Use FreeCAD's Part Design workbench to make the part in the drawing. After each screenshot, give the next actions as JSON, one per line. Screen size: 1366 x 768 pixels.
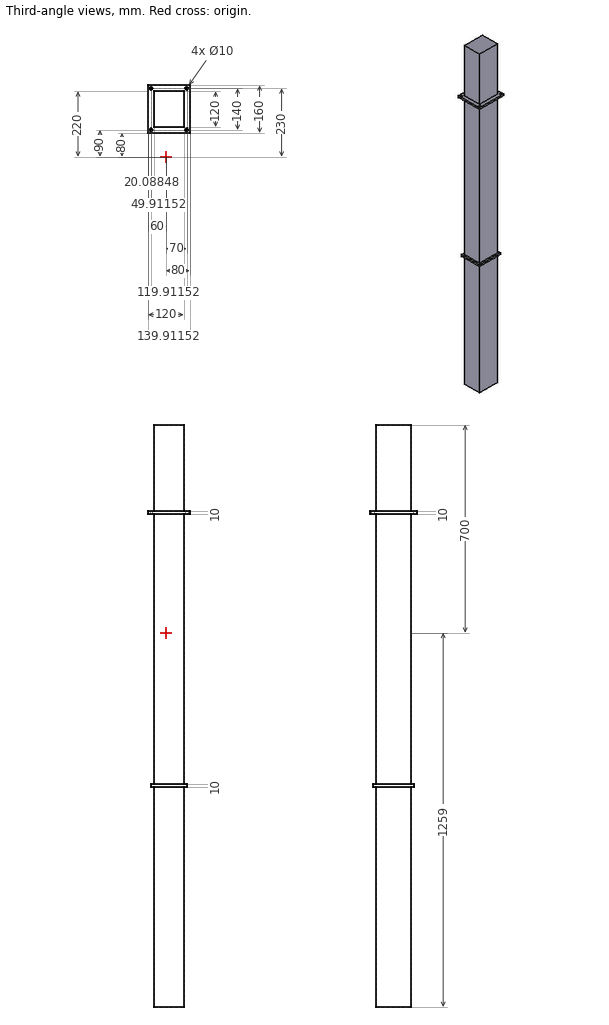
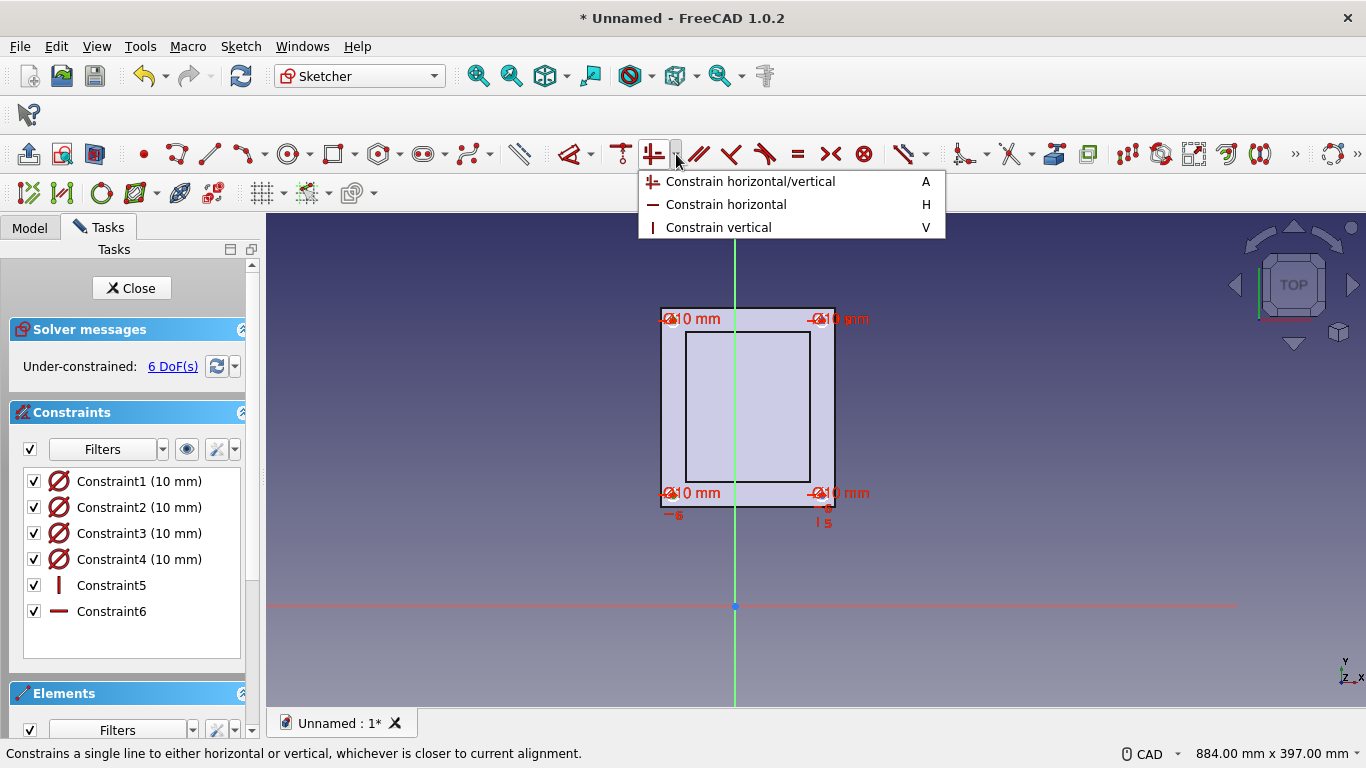
{"action": "left_click", "coordinate": [792, 228]}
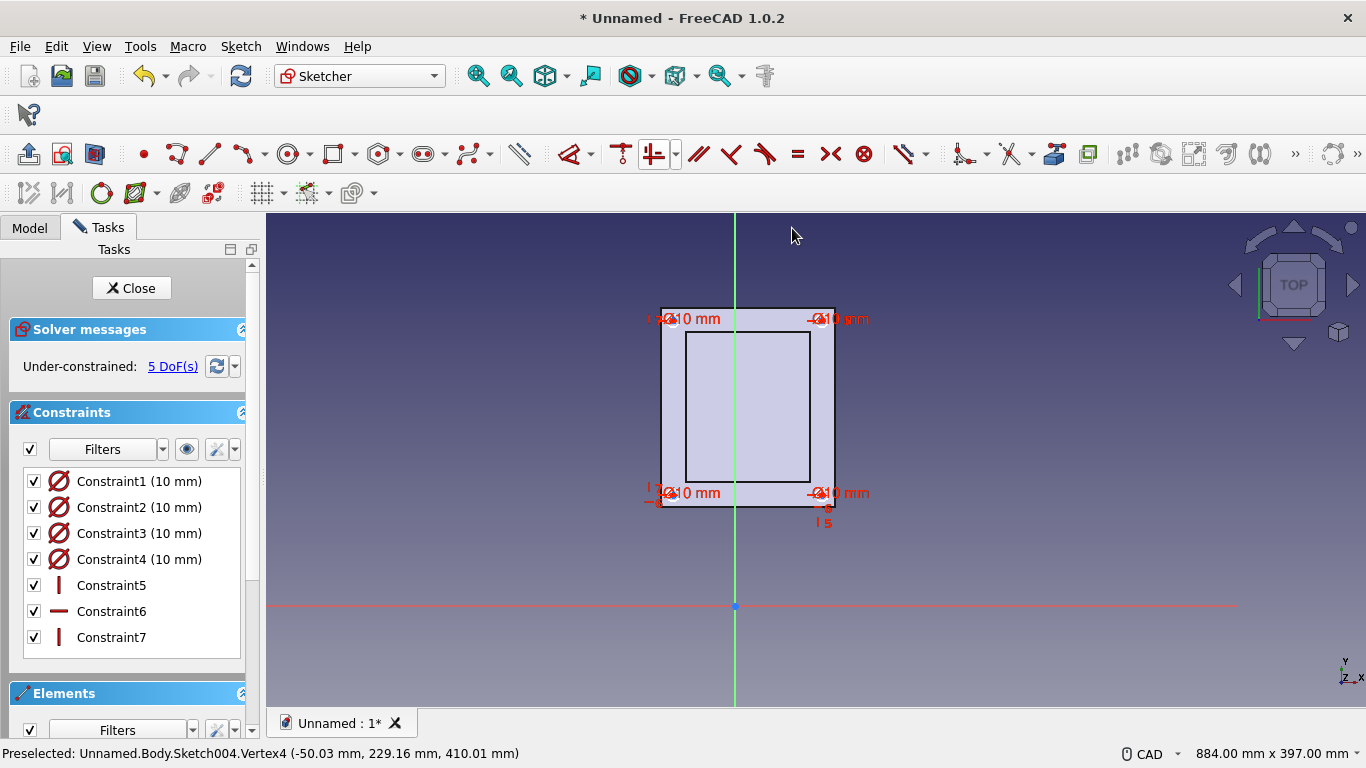
{"action": "left_click", "coordinate": [822, 321]}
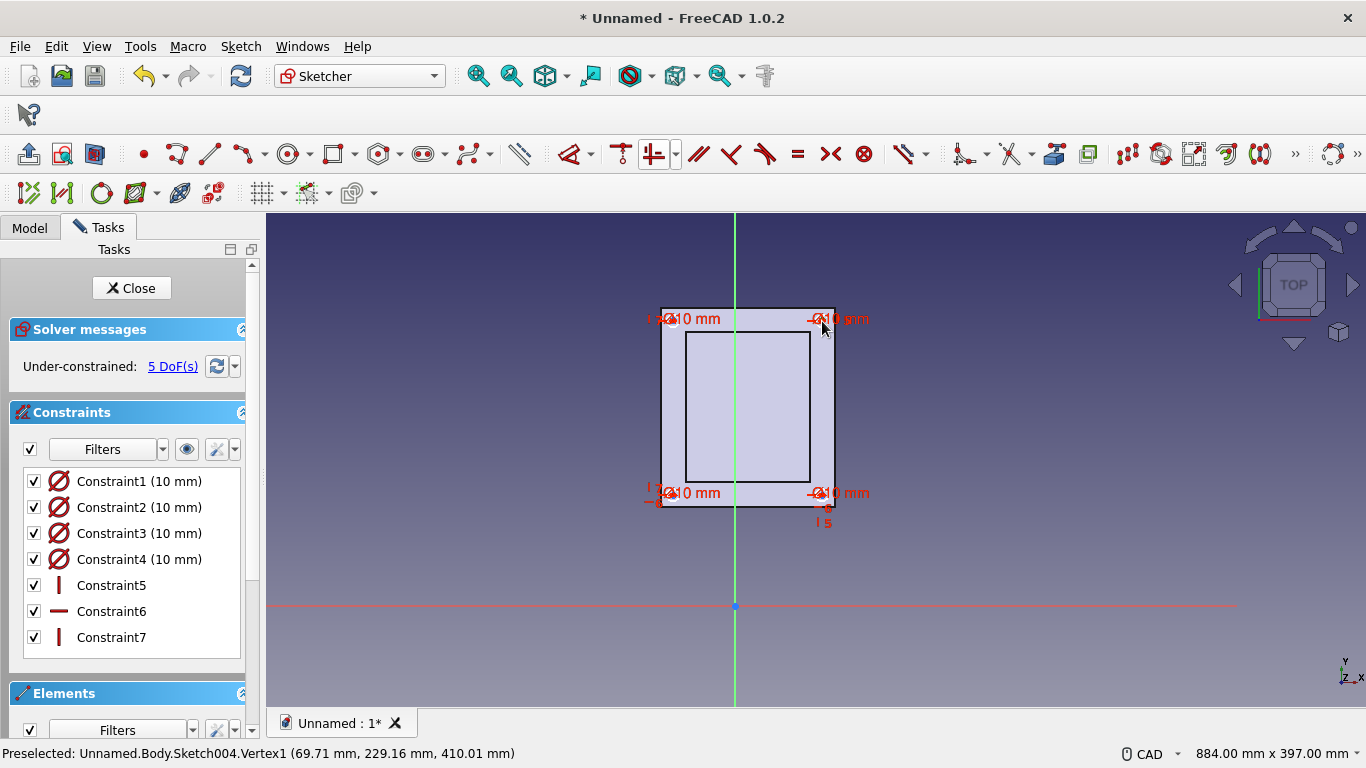
{"action": "left_click", "coordinate": [673, 321]}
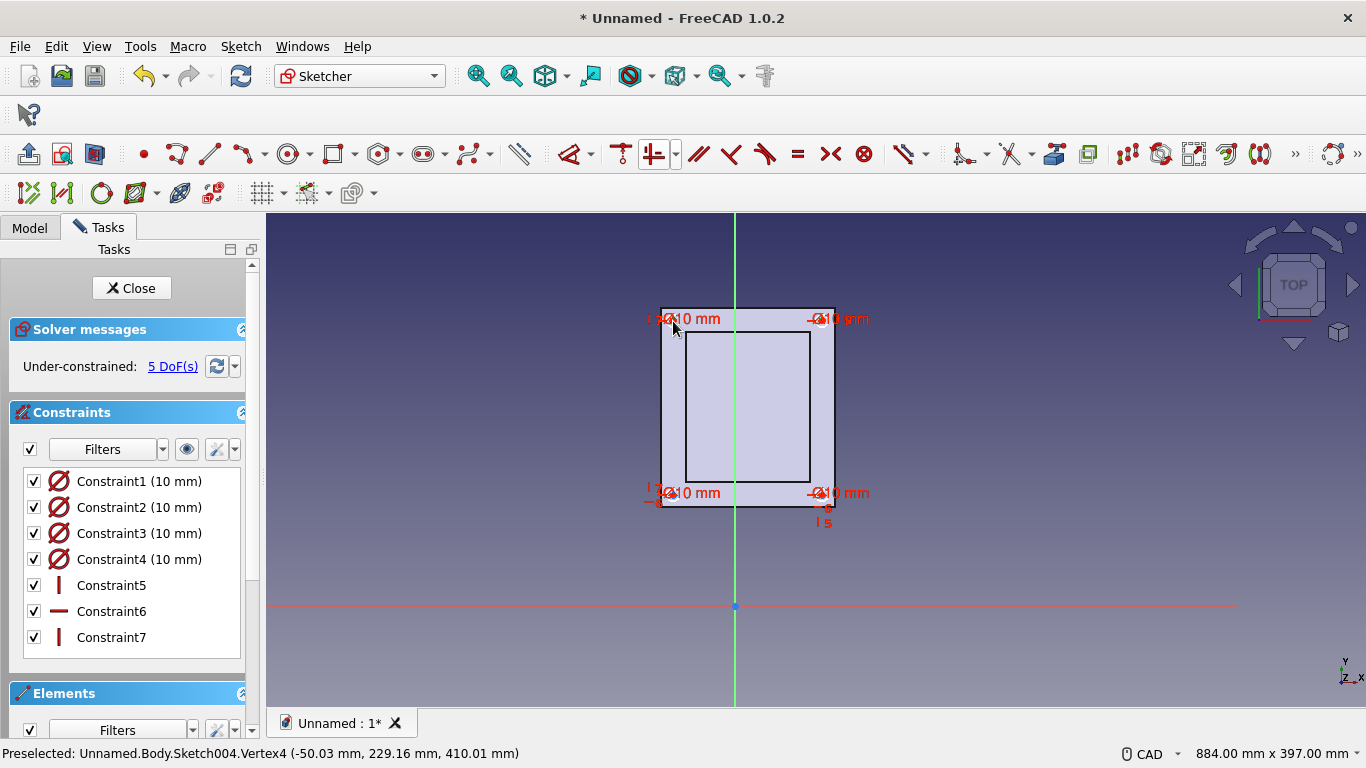
{"action": "key", "text": "h"}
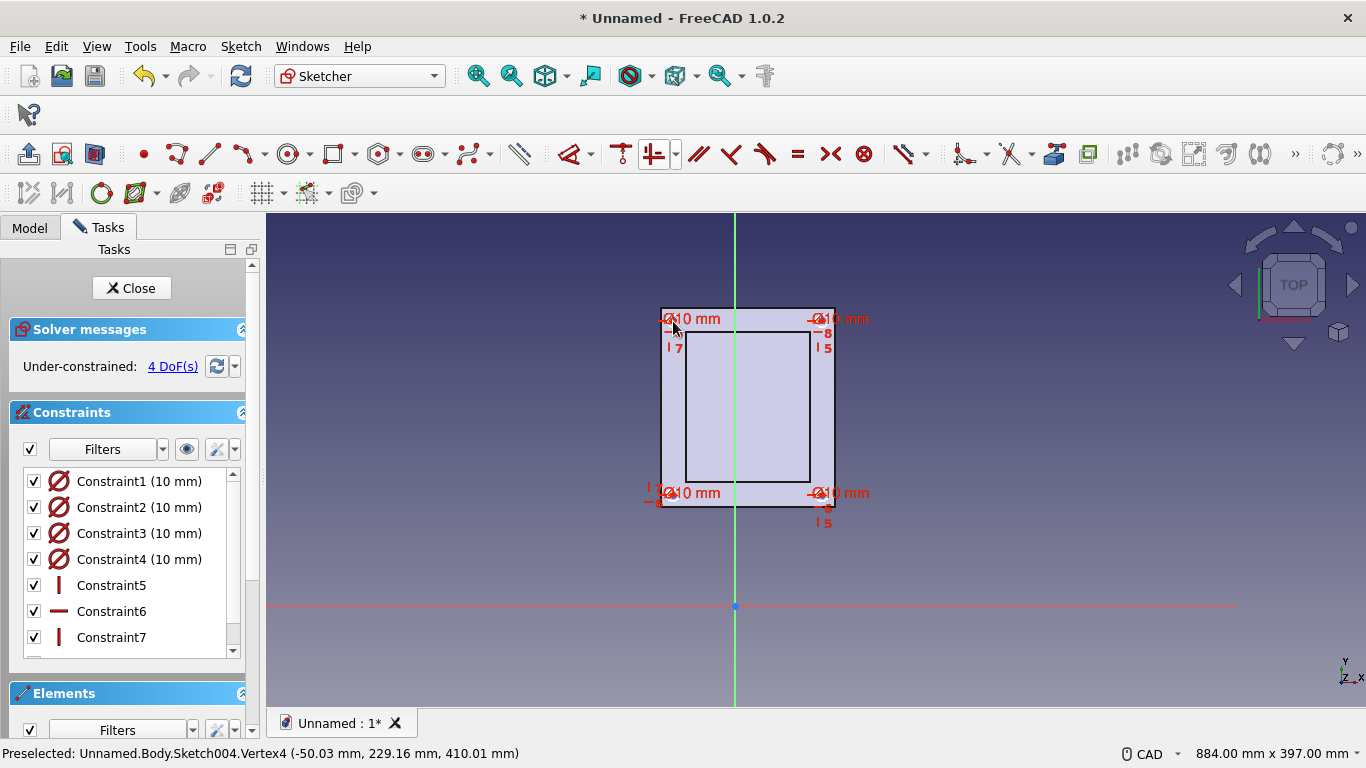
{"action": "key", "text": "d"}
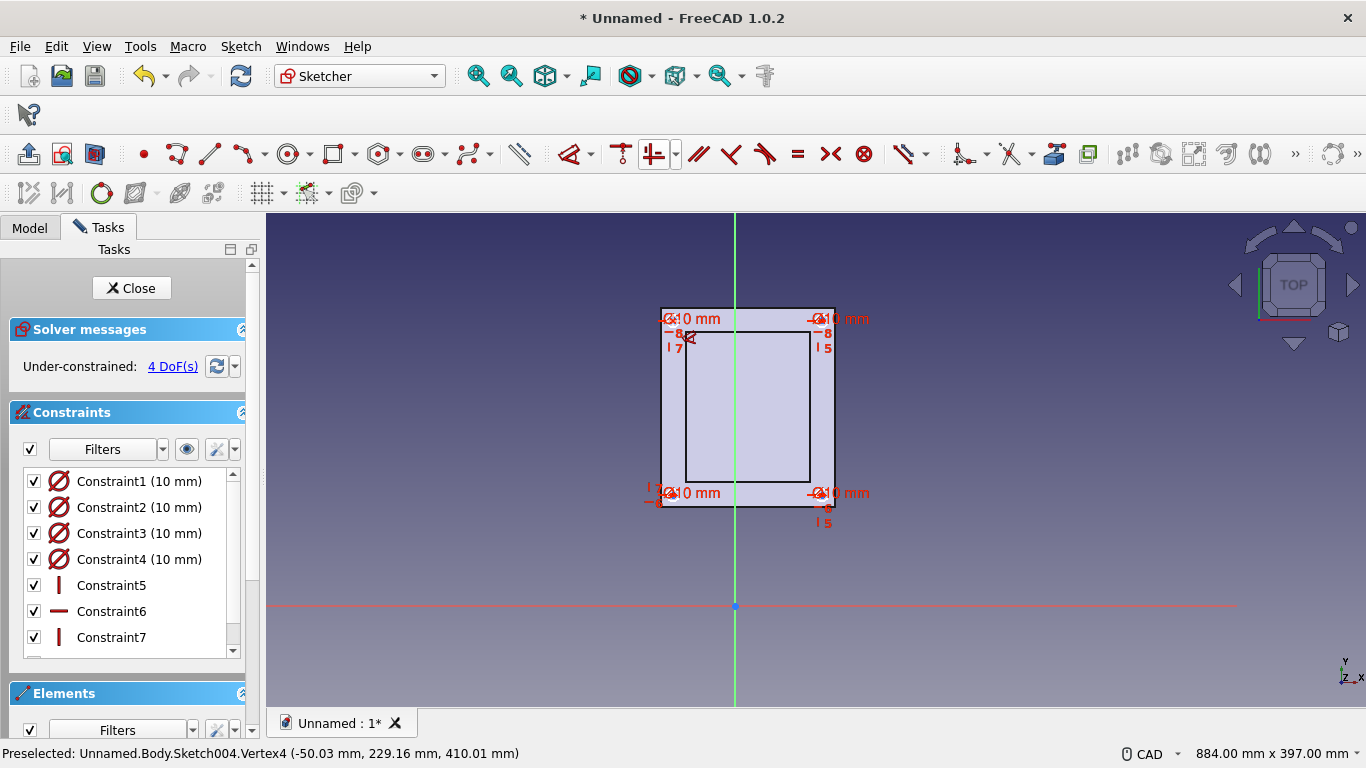
{"action": "left_click", "coordinate": [822, 321]}
{"action": "left_click", "coordinate": [779, 640]}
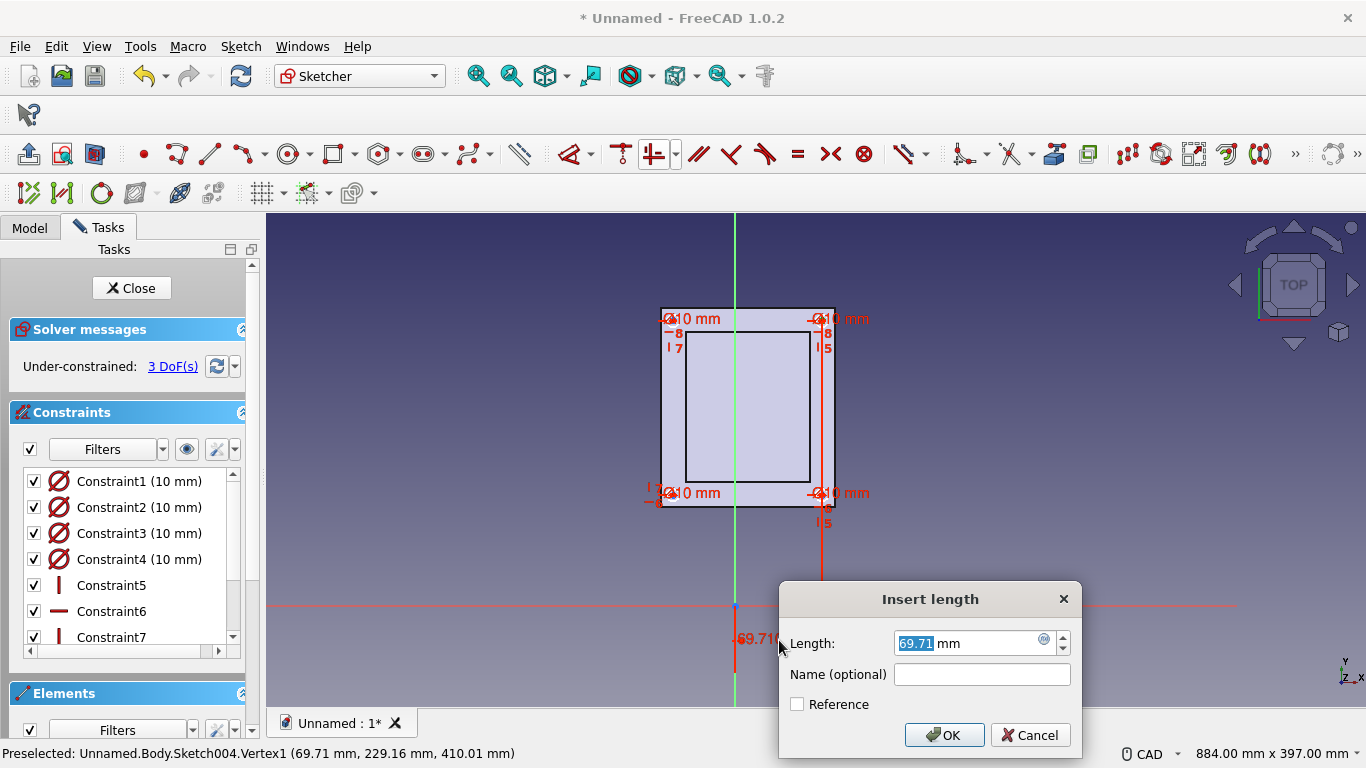
{"action": "type", "text": "70"}
{"action": "key", "text": "Return"}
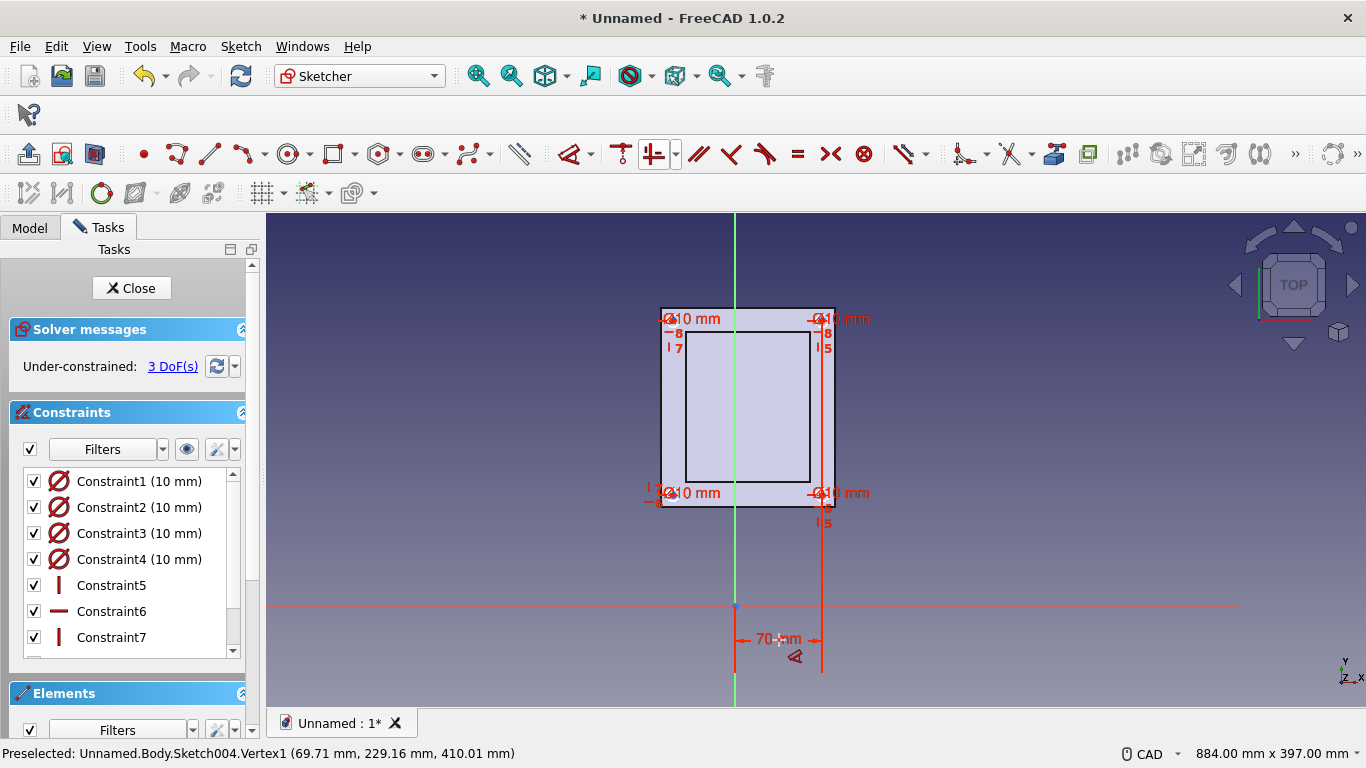
{"action": "left_click", "coordinate": [822, 495]}
{"action": "left_click", "coordinate": [856, 551]}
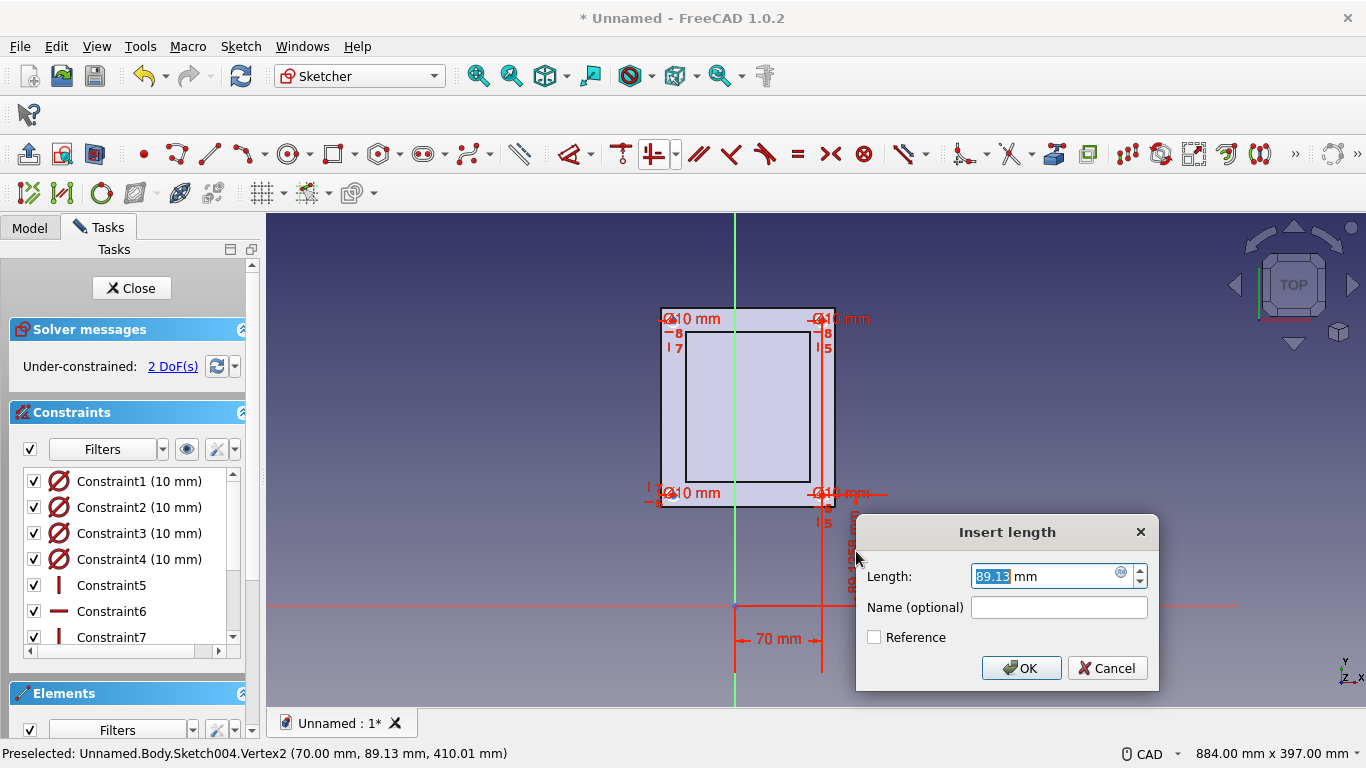
{"action": "type", "text": "90"}
{"action": "key", "text": "Return"}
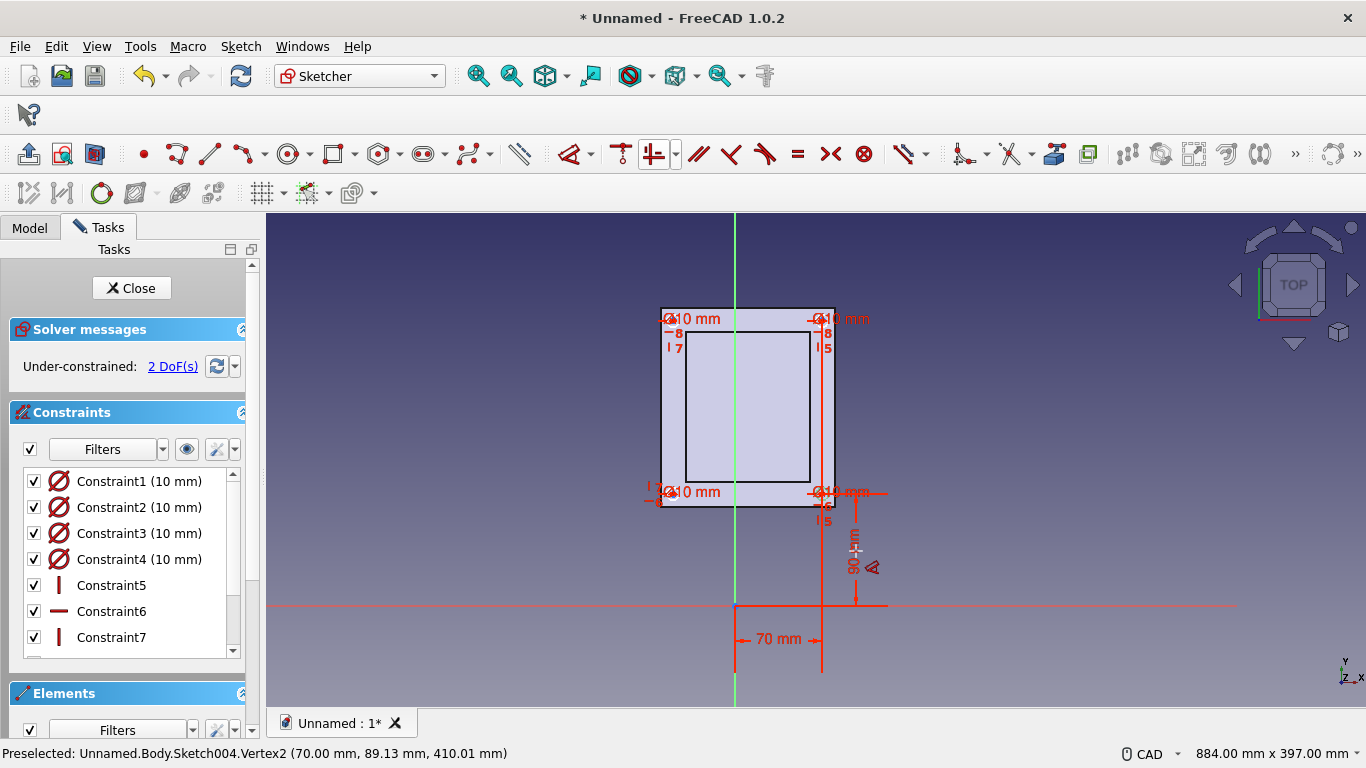
{"action": "left_click", "coordinate": [822, 321]}
{"action": "left_click", "coordinate": [856, 464]}